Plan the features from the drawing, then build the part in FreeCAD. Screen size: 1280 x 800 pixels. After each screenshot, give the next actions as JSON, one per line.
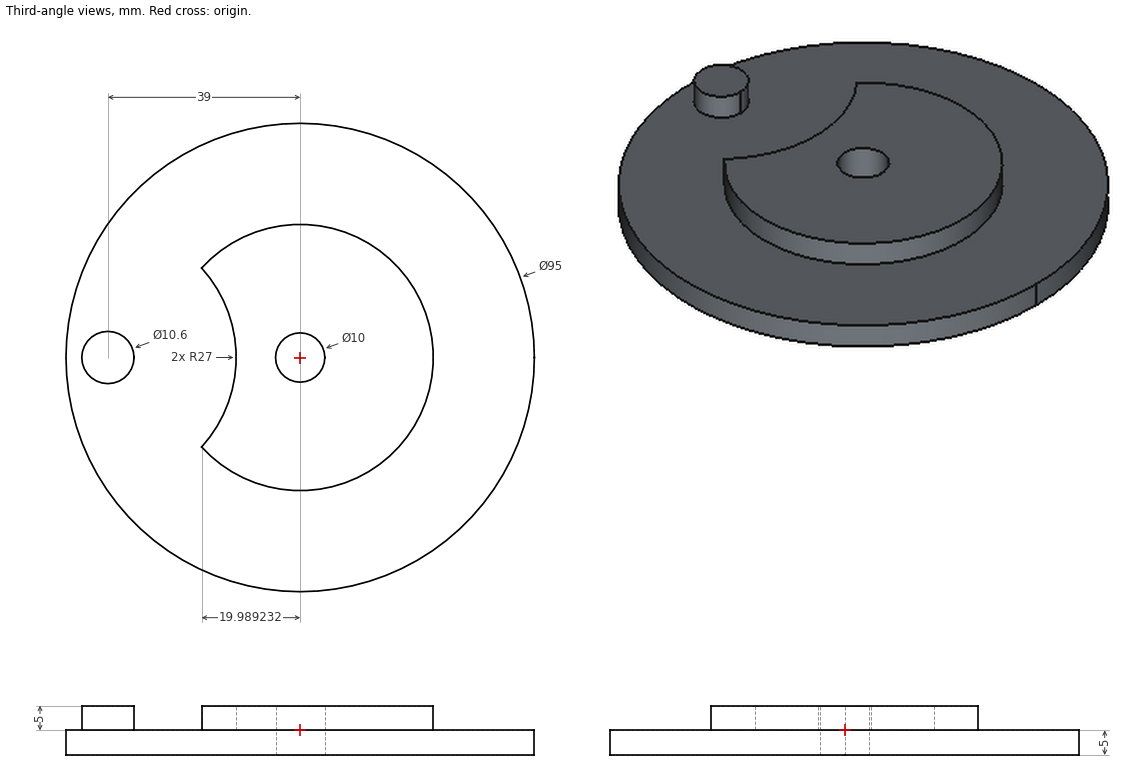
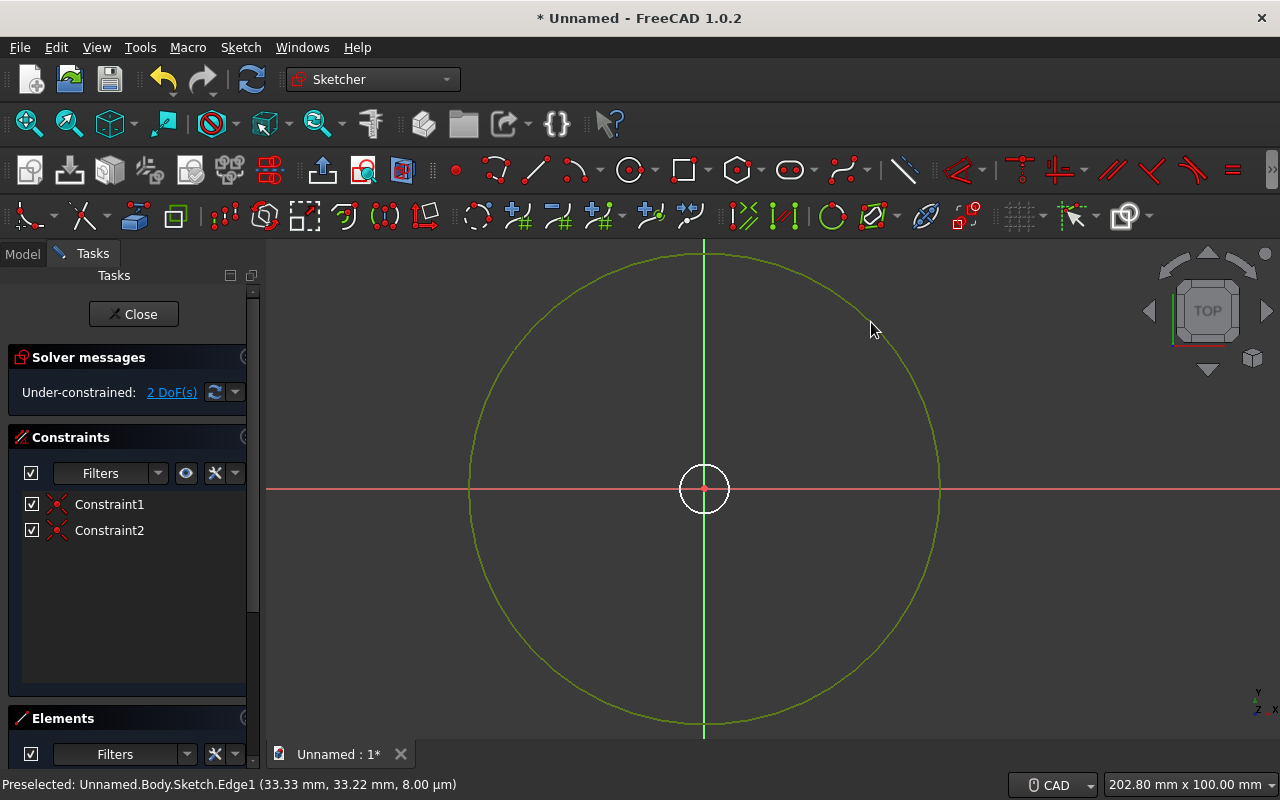
{"action": "left_click", "coordinate": [984, 170]}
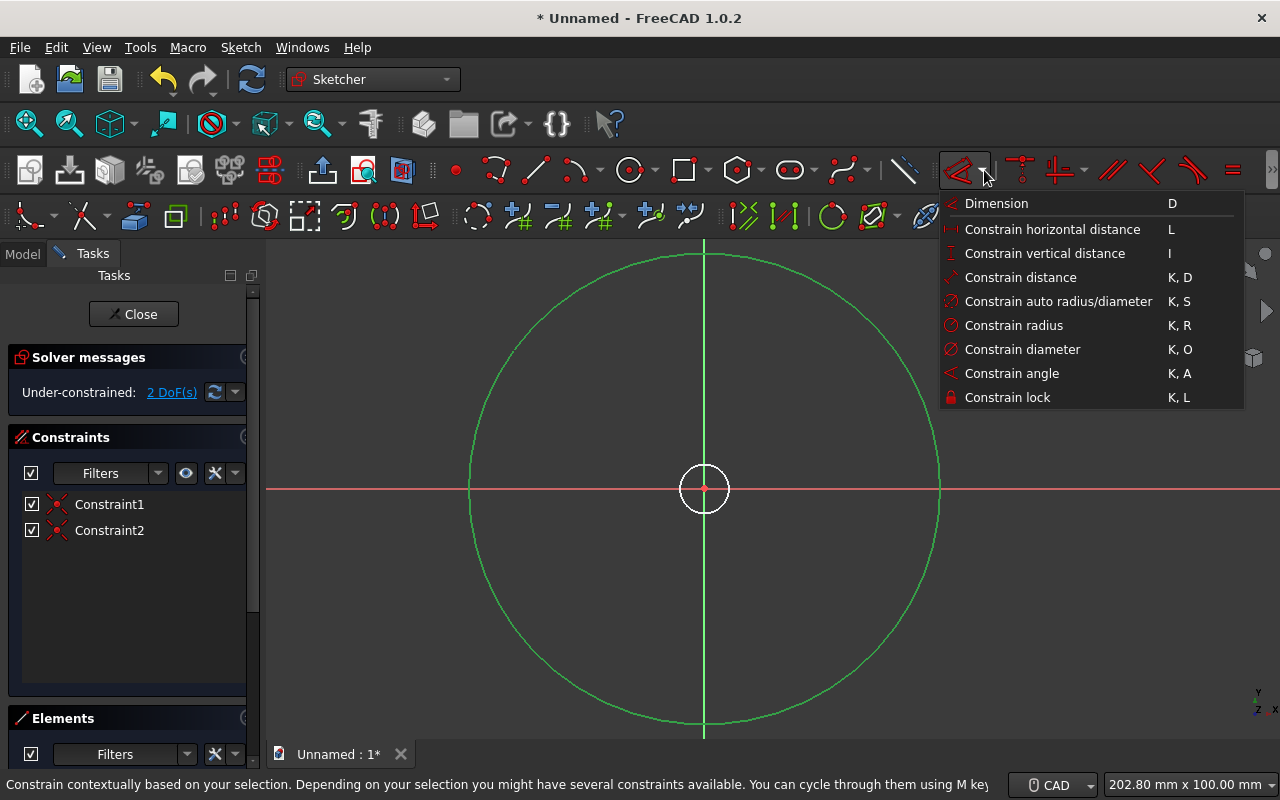
{"action": "left_click", "coordinate": [1092, 349]}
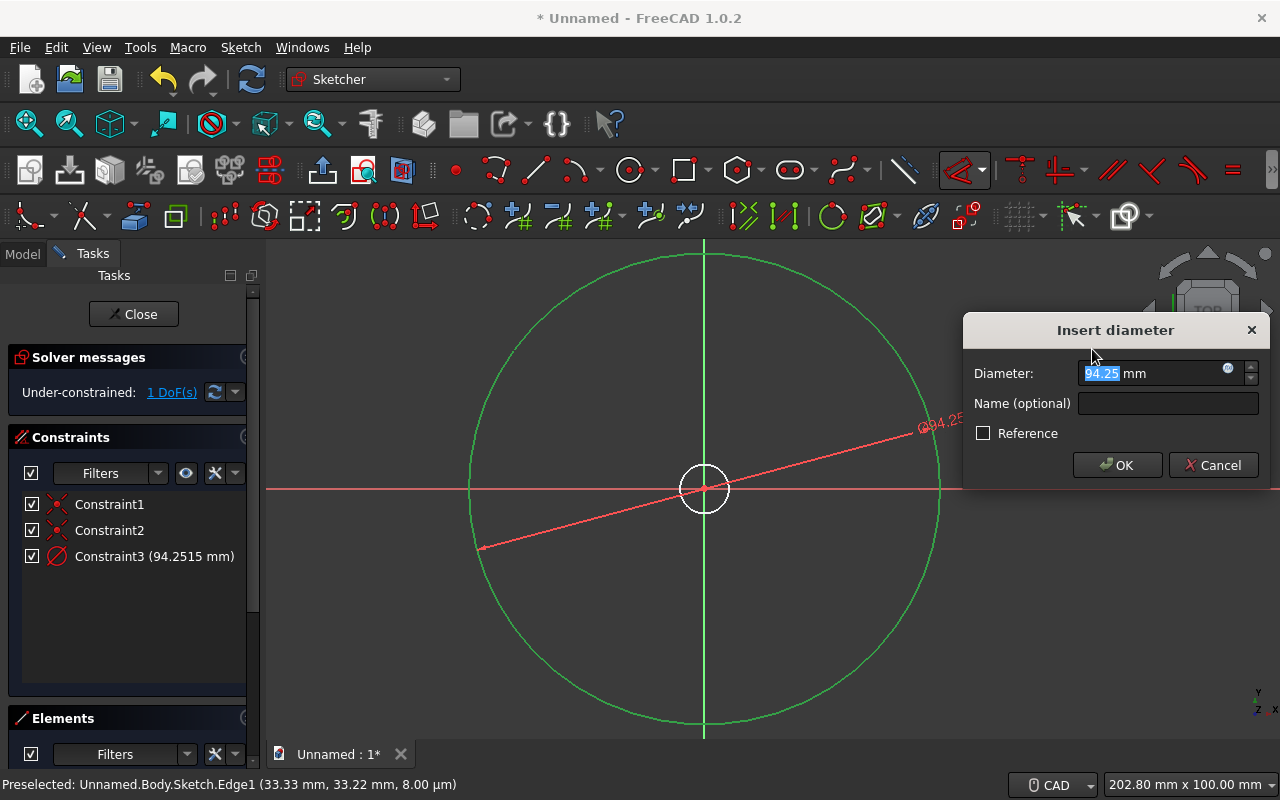
{"action": "type", "text": "95"}
{"action": "key", "text": "Return"}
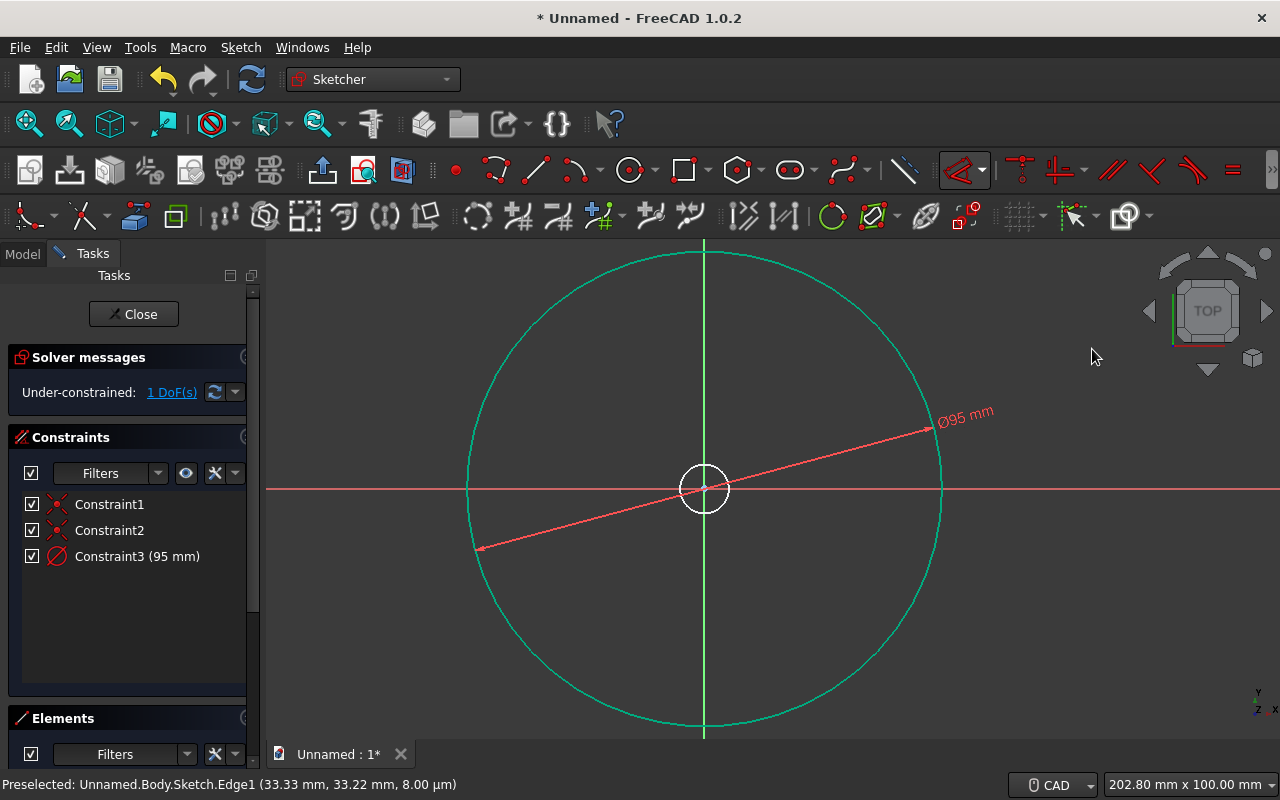
{"action": "left_click", "coordinate": [722, 472]}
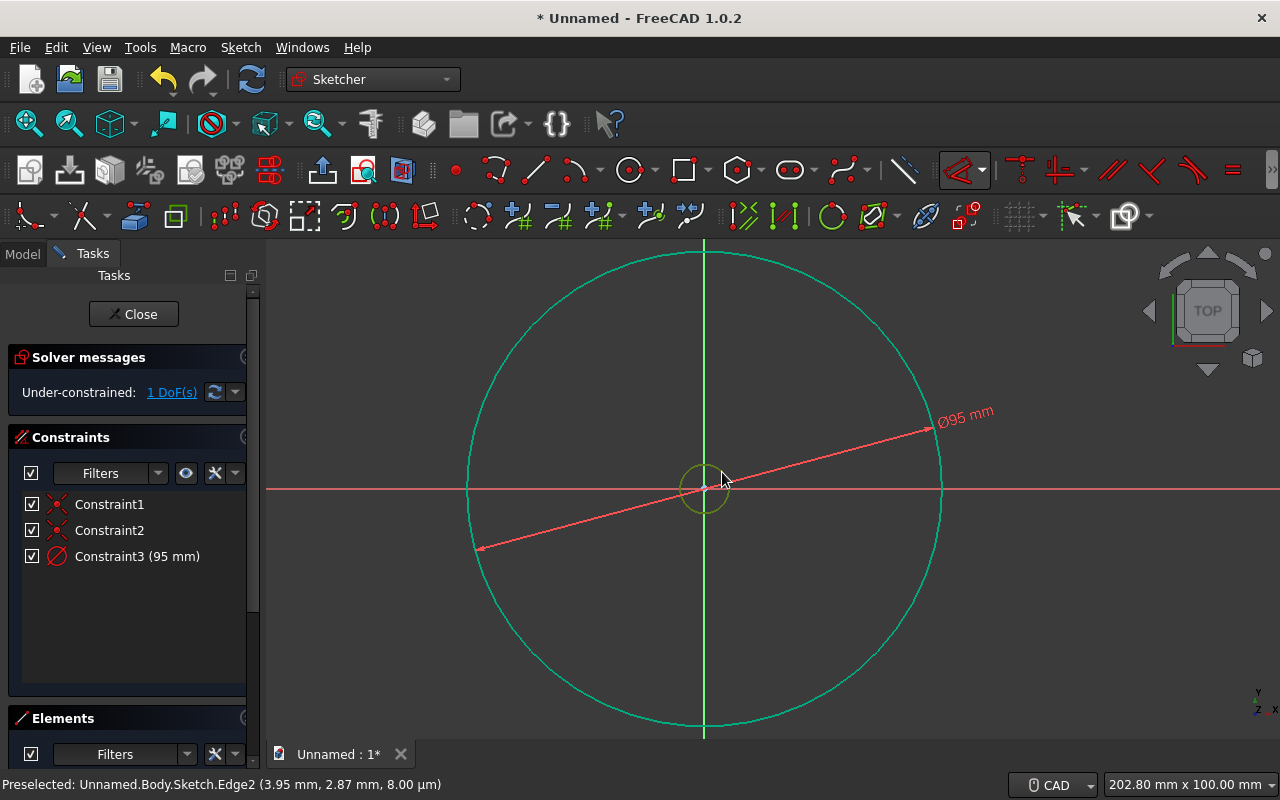
{"action": "left_click", "coordinate": [984, 170]}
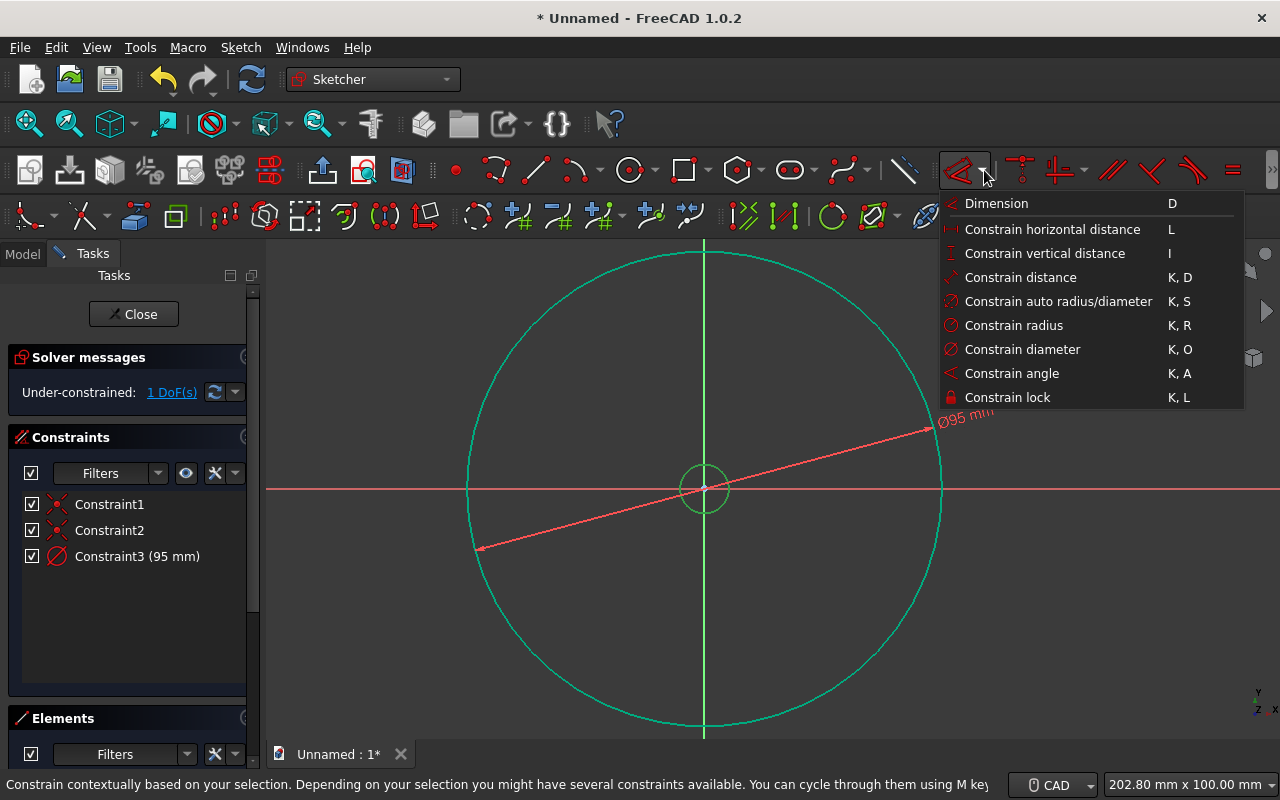
{"action": "left_click", "coordinate": [1092, 349]}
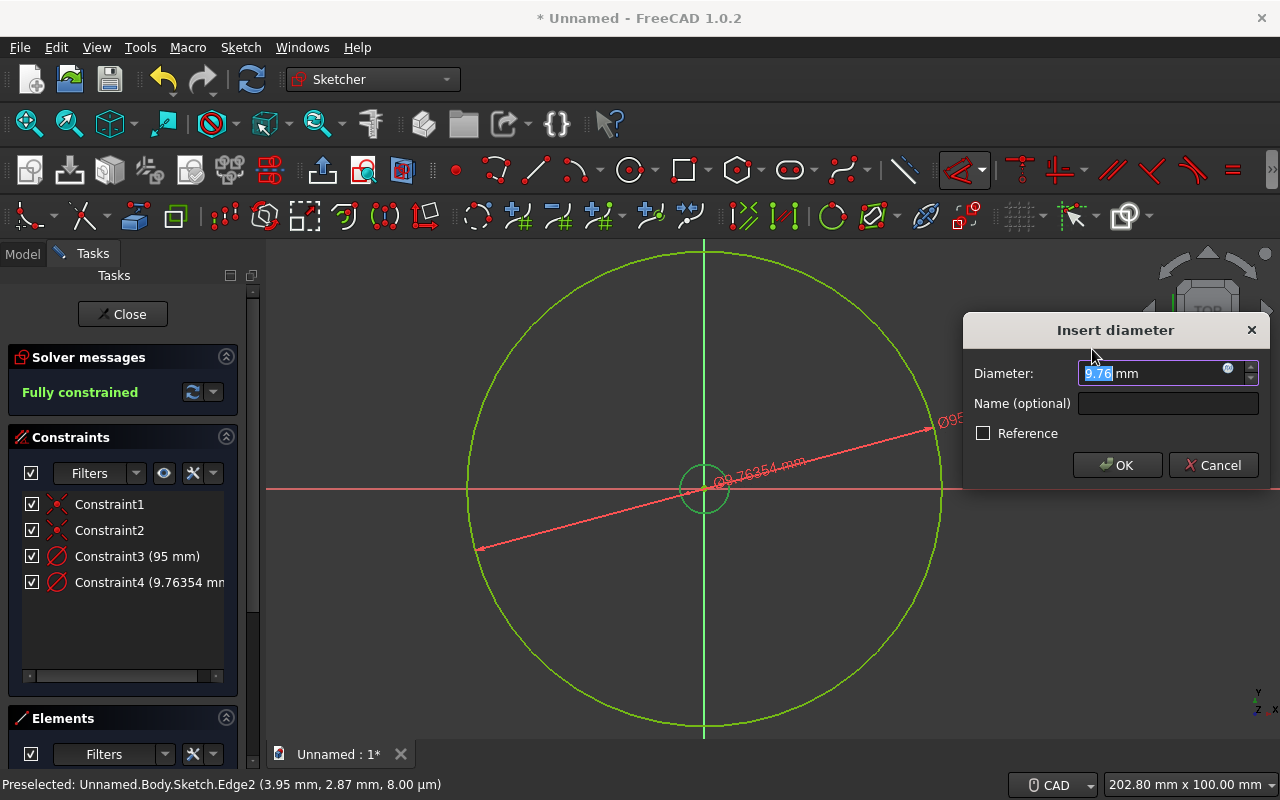
{"action": "type", "text": "10"}
{"action": "key", "text": "Return"}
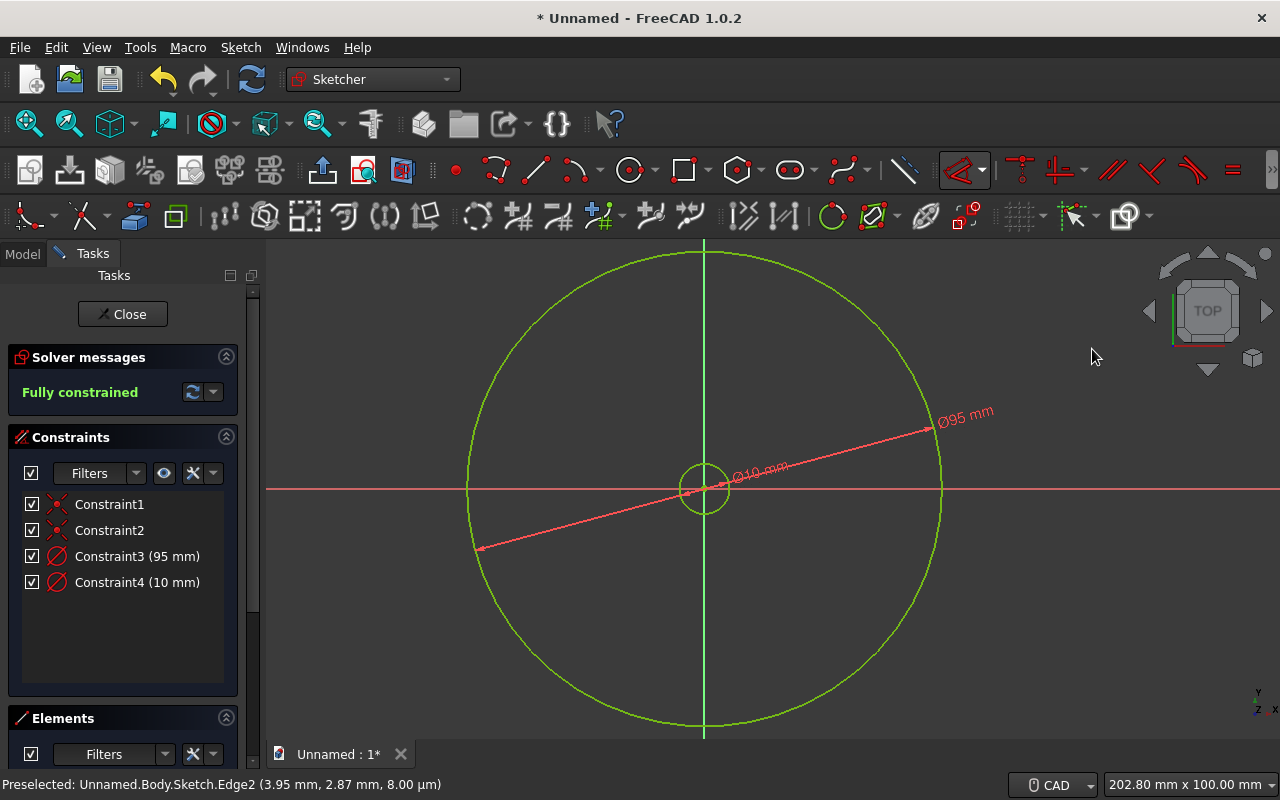
{"action": "left_click", "coordinate": [123, 314]}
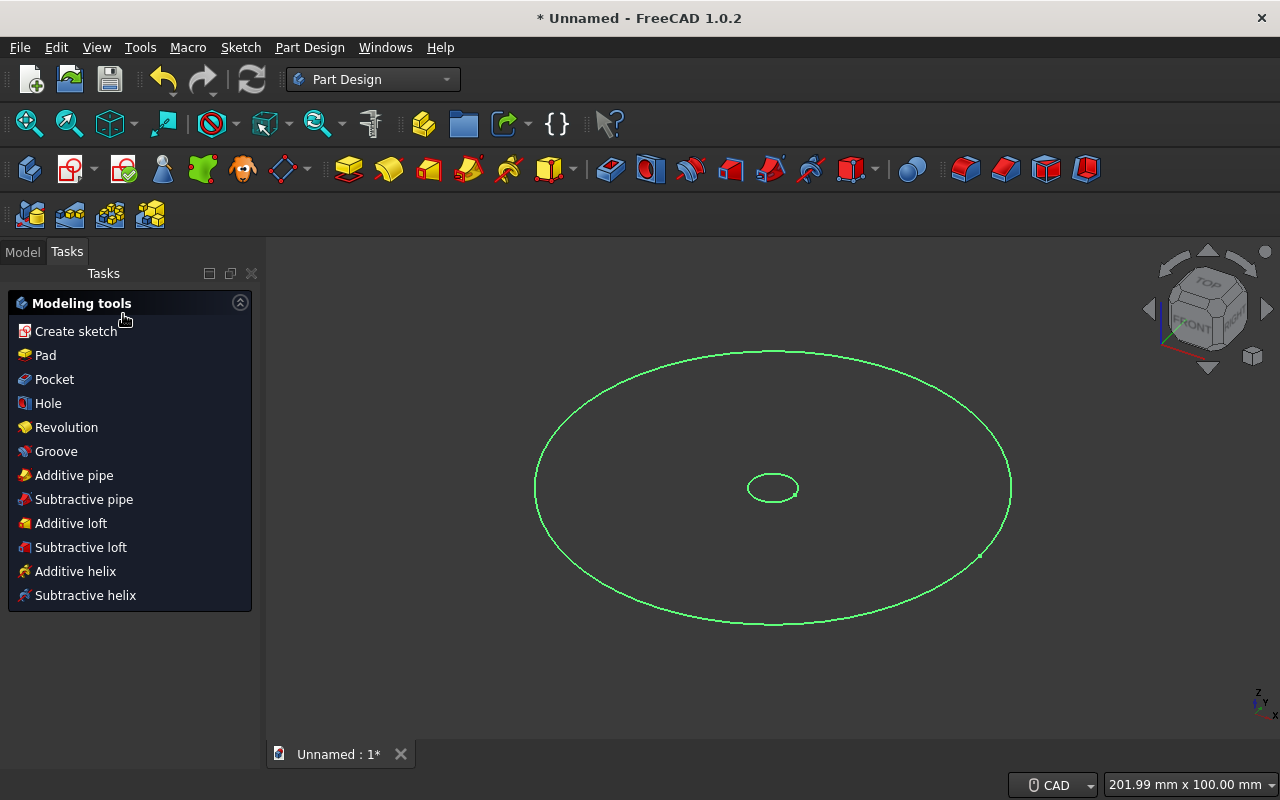
{"action": "left_click", "coordinate": [350, 170]}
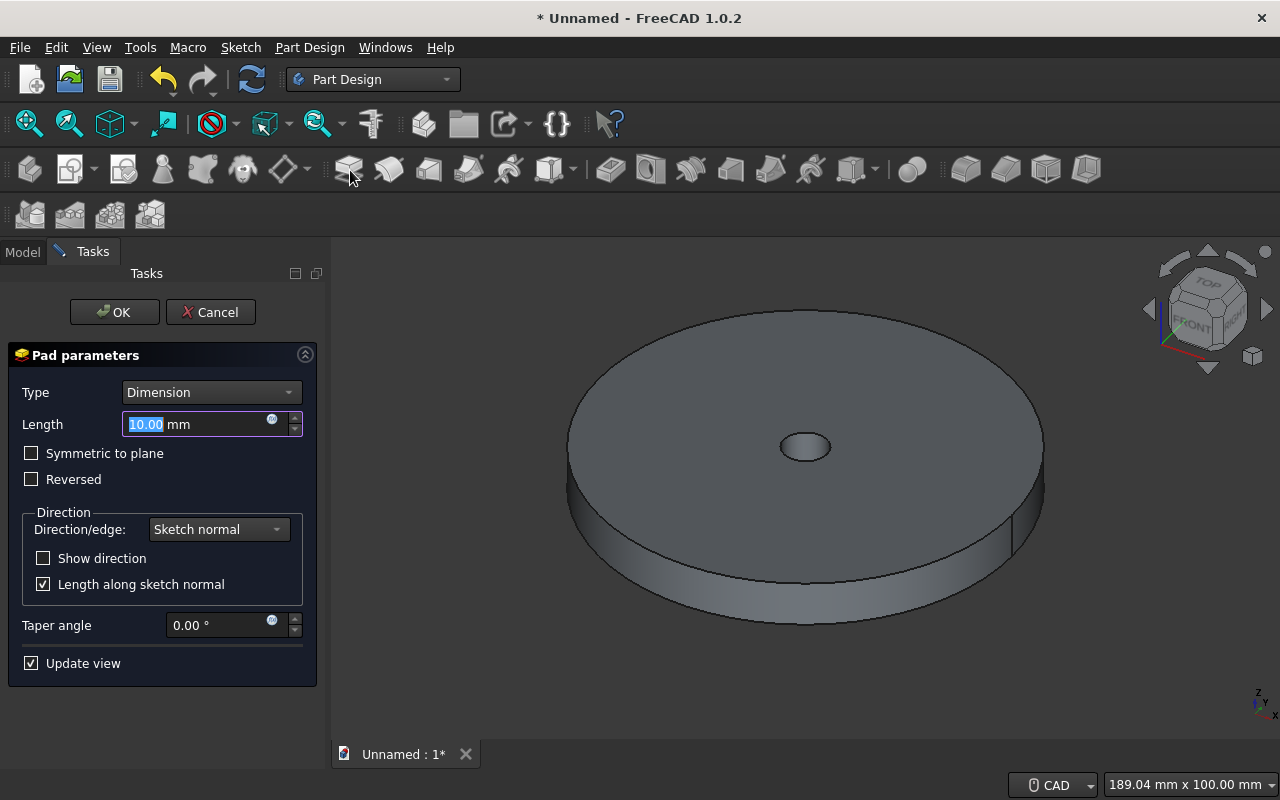
{"action": "type", "text": "5"}
{"action": "key", "text": "Tab"}